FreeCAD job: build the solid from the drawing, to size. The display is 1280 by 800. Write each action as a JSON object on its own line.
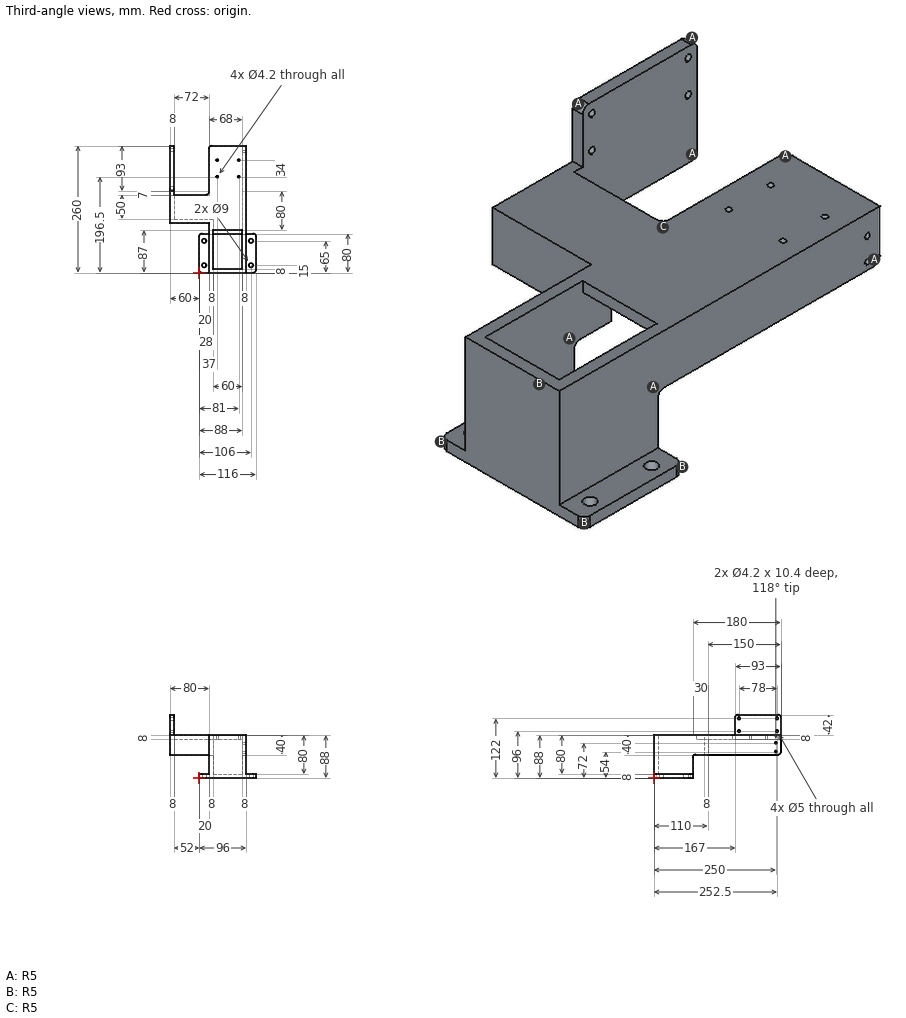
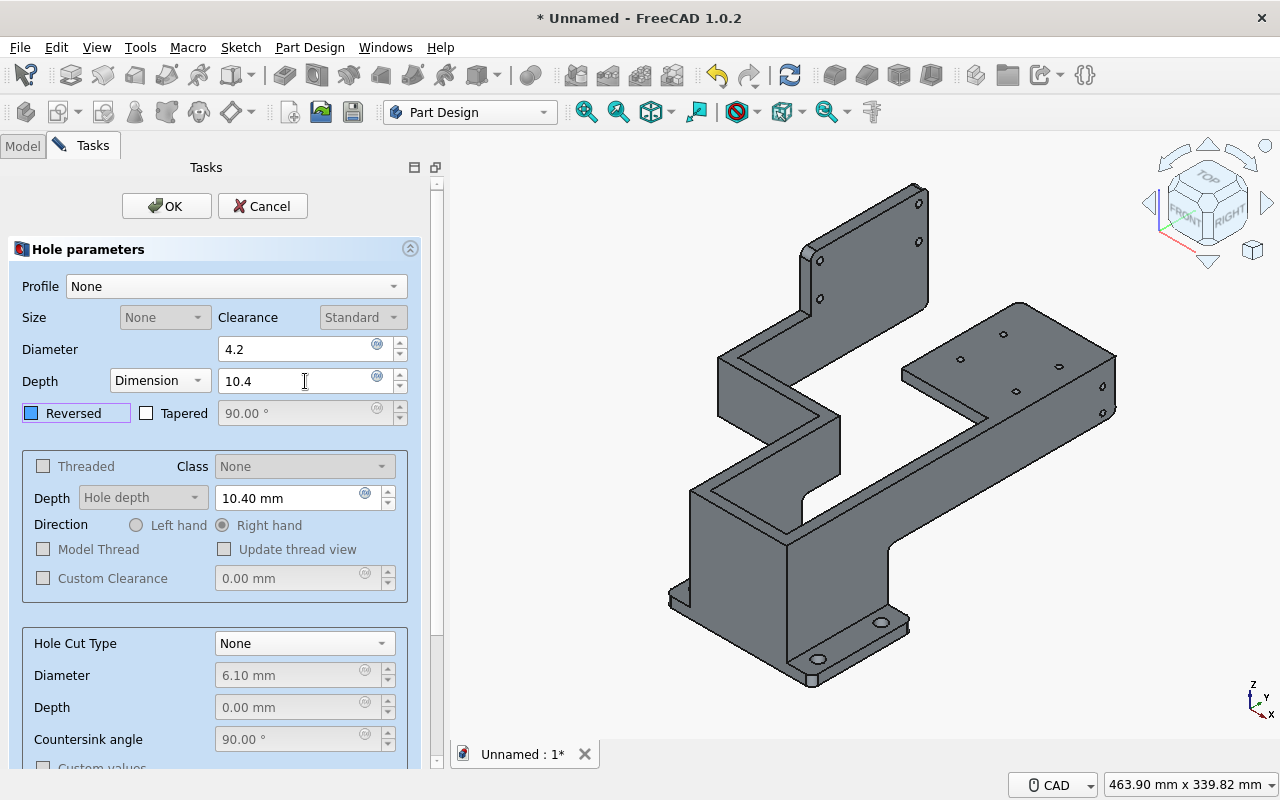
{"action": "left_click", "coordinate": [167, 206]}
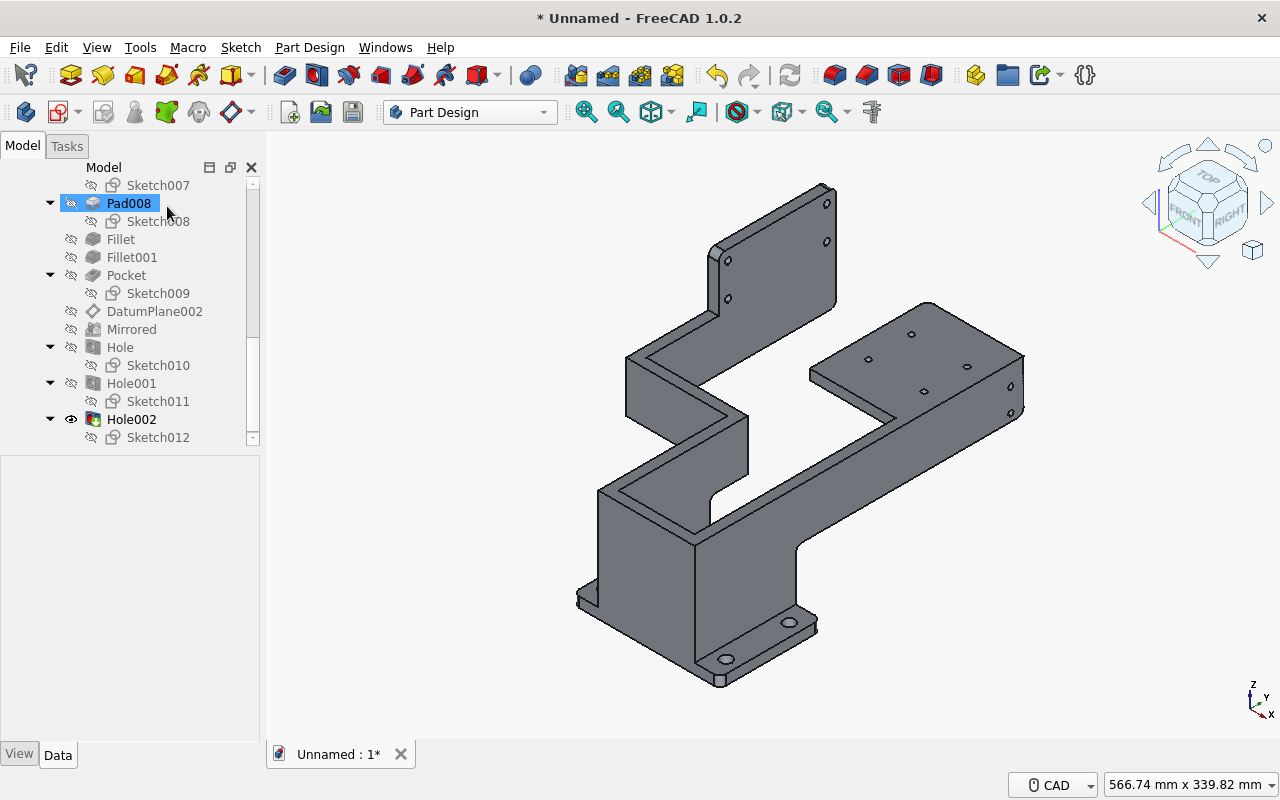
{"action": "left_click", "coordinate": [958, 344]}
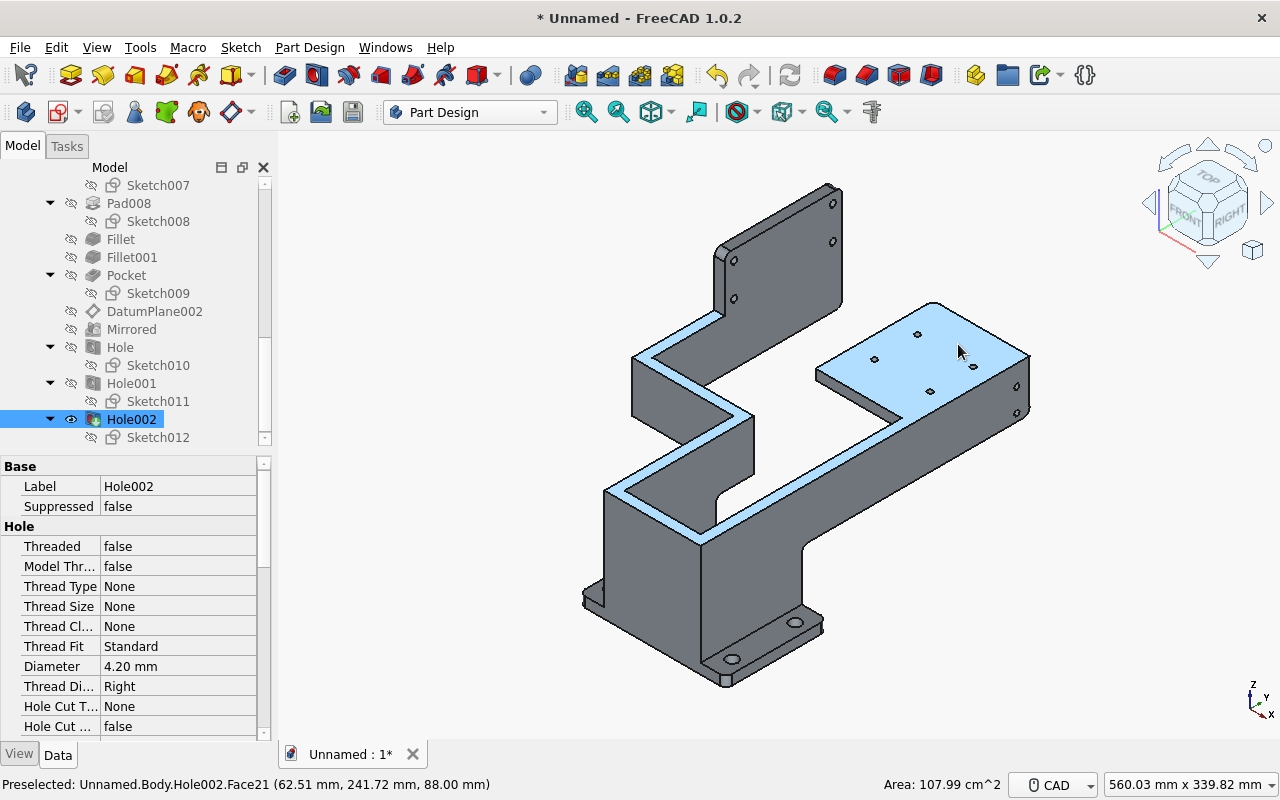
{"action": "left_click", "coordinate": [58, 112]}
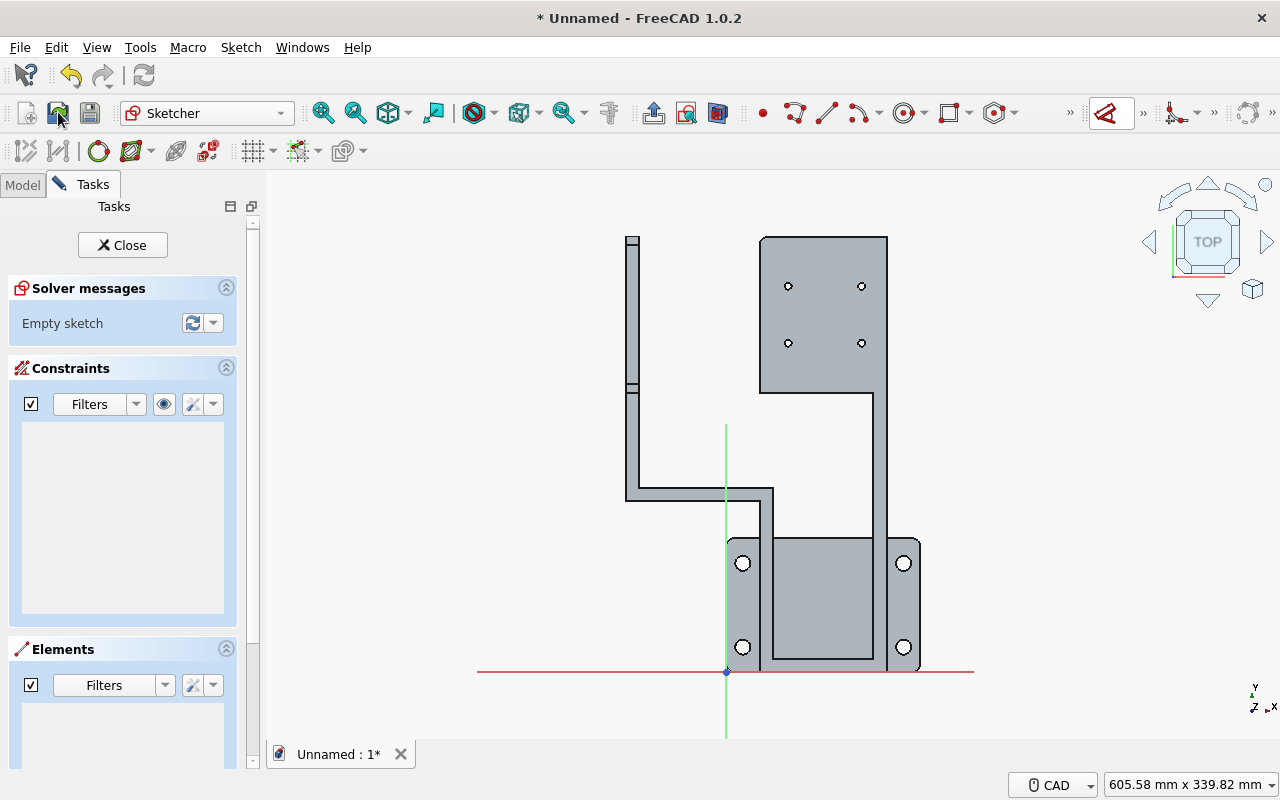
{"action": "left_click", "coordinate": [796, 114]}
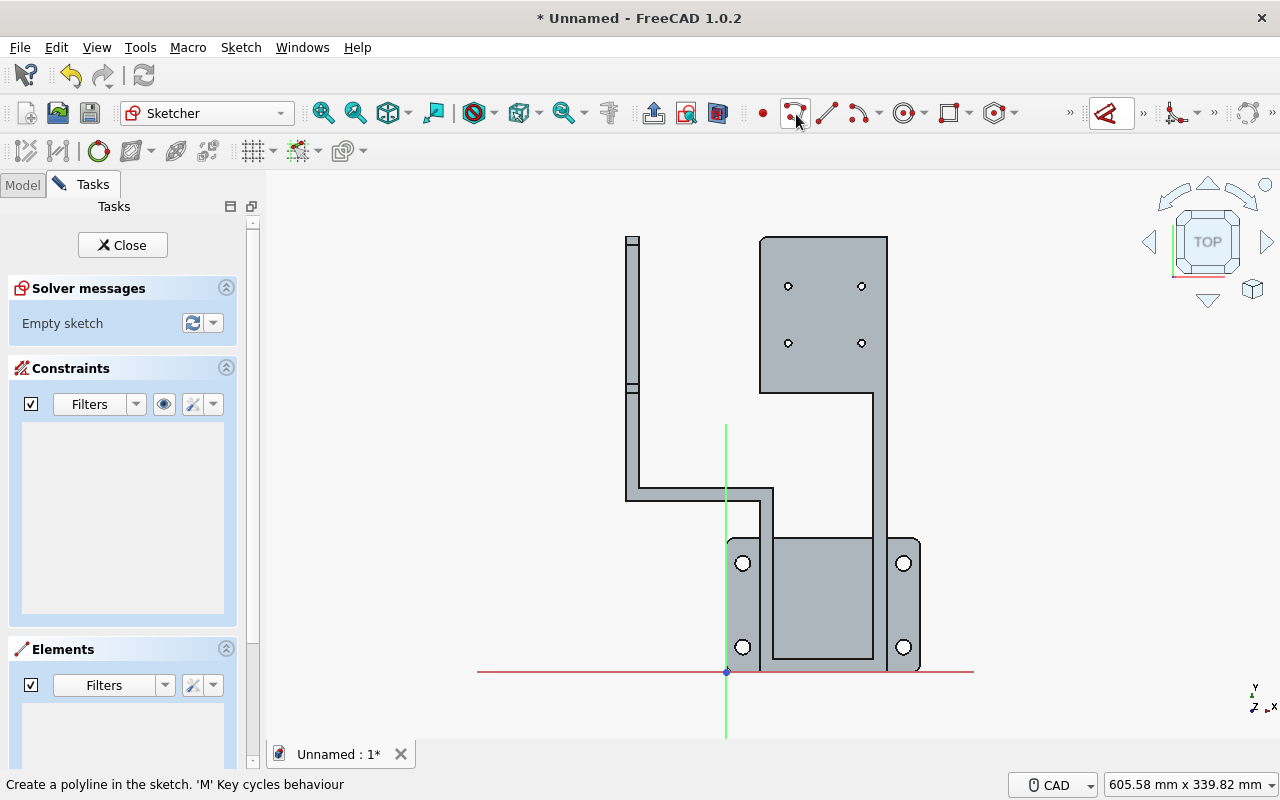
{"action": "left_click", "coordinate": [773, 527]}
{"action": "left_click", "coordinate": [873, 527]}
{"action": "left_click", "coordinate": [873, 393]}
{"action": "left_click", "coordinate": [760, 393]}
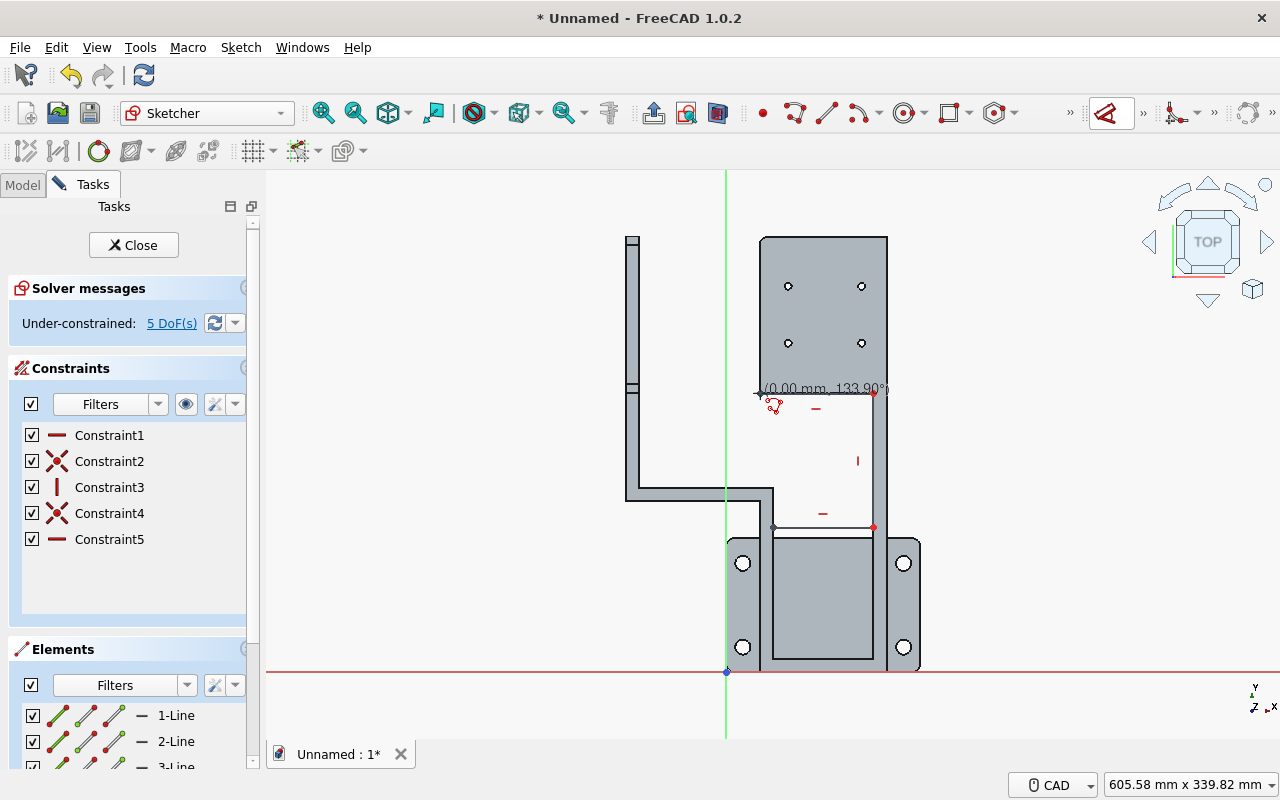
{"action": "scroll", "coordinate": [760, 404], "scroll_direction": "up", "scroll_amount": 2}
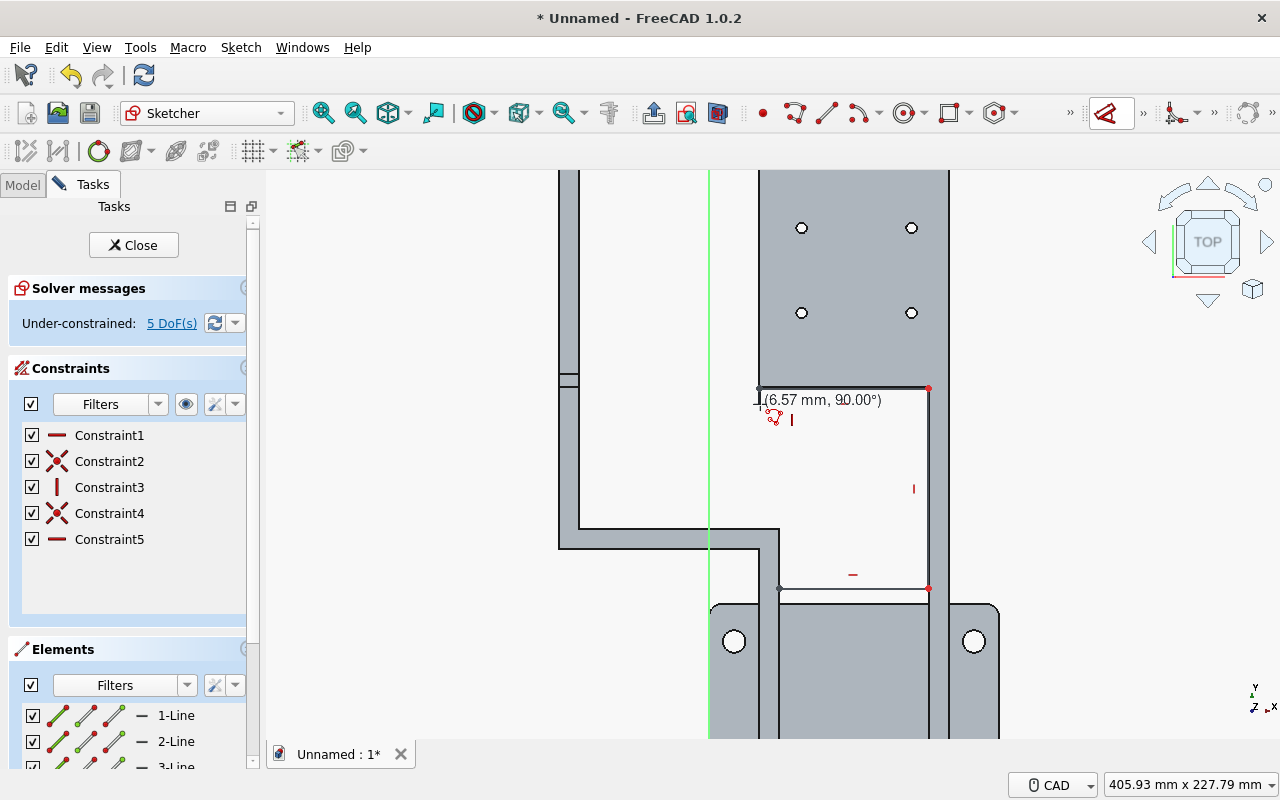
{"action": "left_click", "coordinate": [760, 404]}
{"action": "left_click", "coordinate": [579, 404]}
{"action": "left_click", "coordinate": [579, 529]}
{"action": "left_click", "coordinate": [779, 529]}
{"action": "left_click", "coordinate": [779, 589]}
{"action": "key", "text": "Escape"}
{"action": "key", "text": "Escape"}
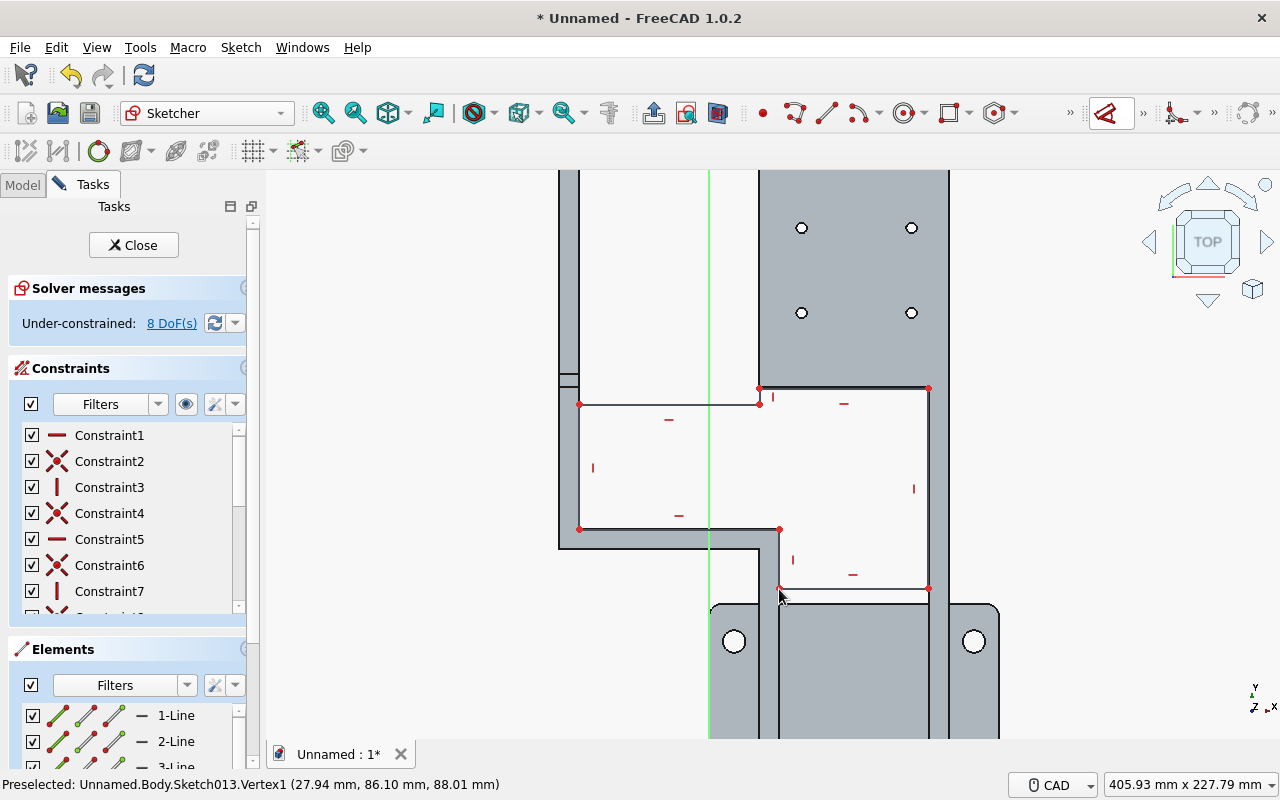
{"action": "scroll", "coordinate": [760, 397], "scroll_direction": "up", "scroll_amount": 5}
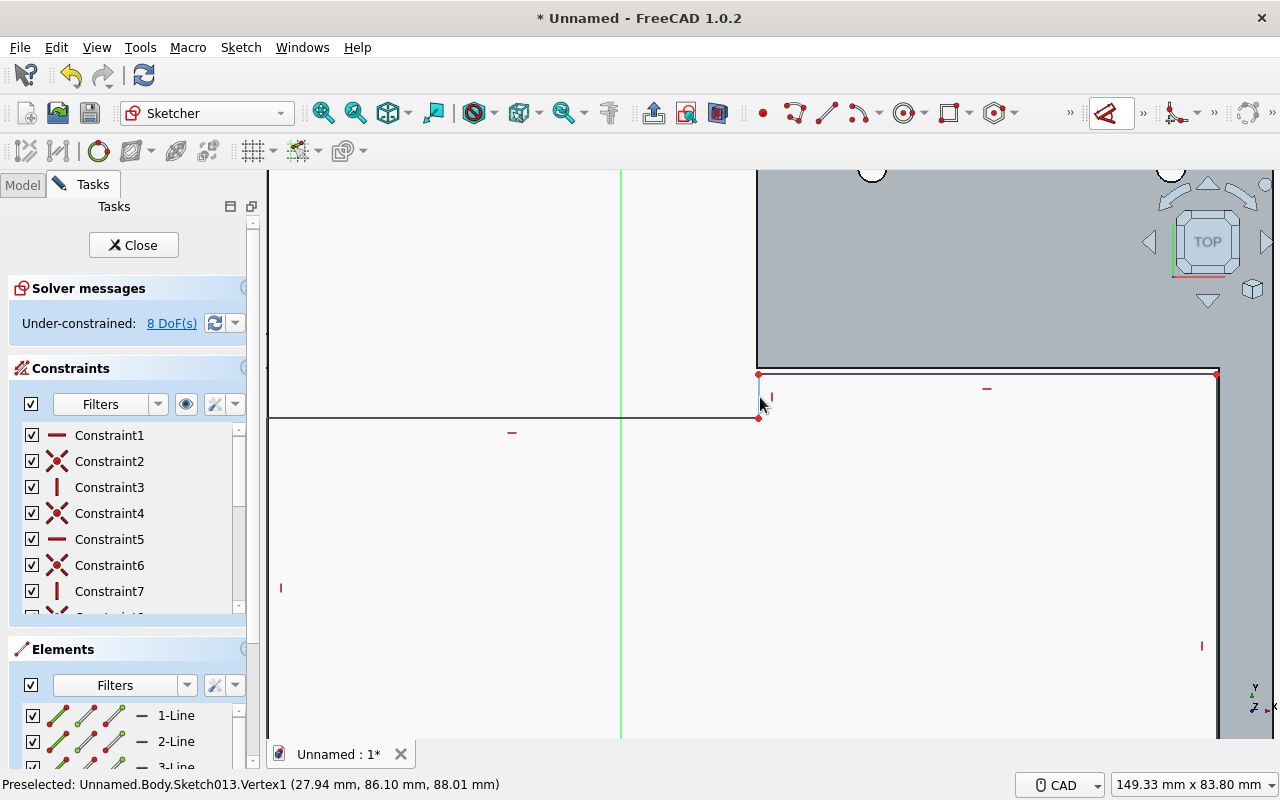
{"action": "left_click", "coordinate": [759, 396]}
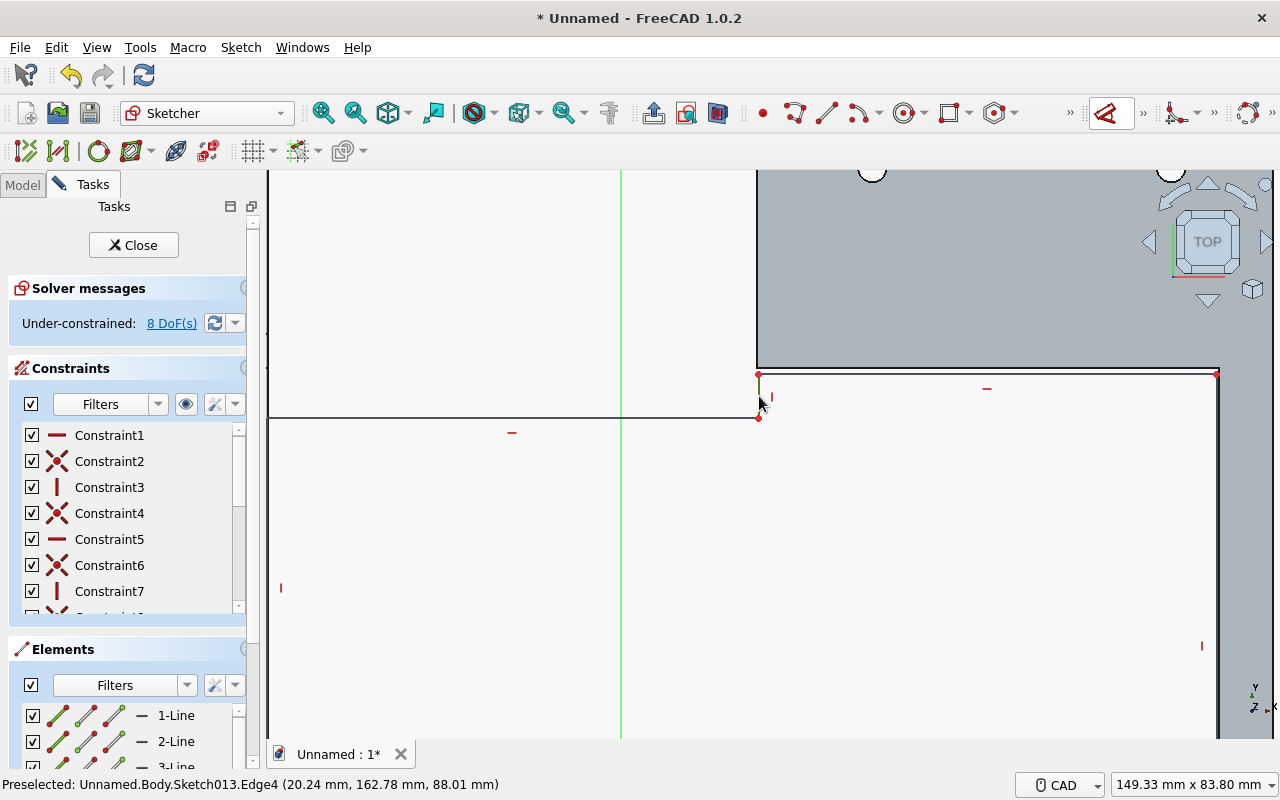
{"action": "left_click", "coordinate": [1128, 114]}